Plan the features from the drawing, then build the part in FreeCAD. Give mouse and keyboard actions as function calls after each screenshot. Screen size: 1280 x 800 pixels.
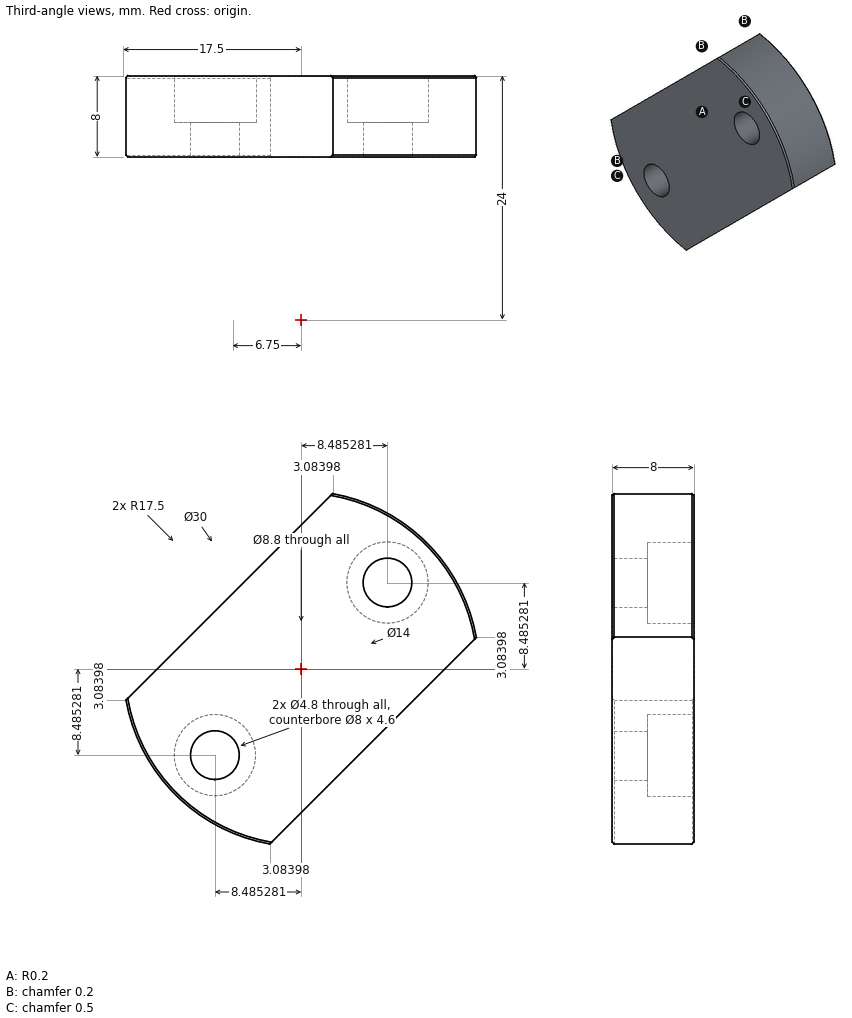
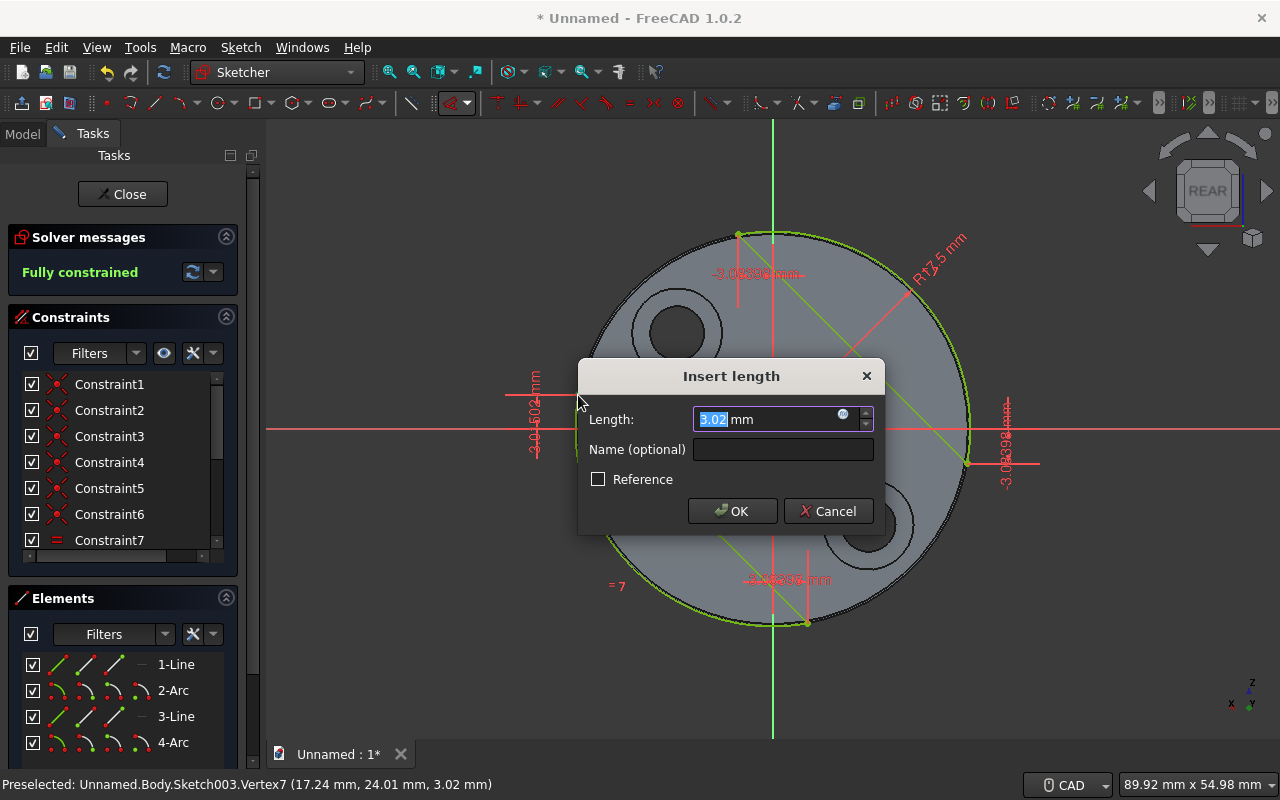
text(3.08398)
key(Return)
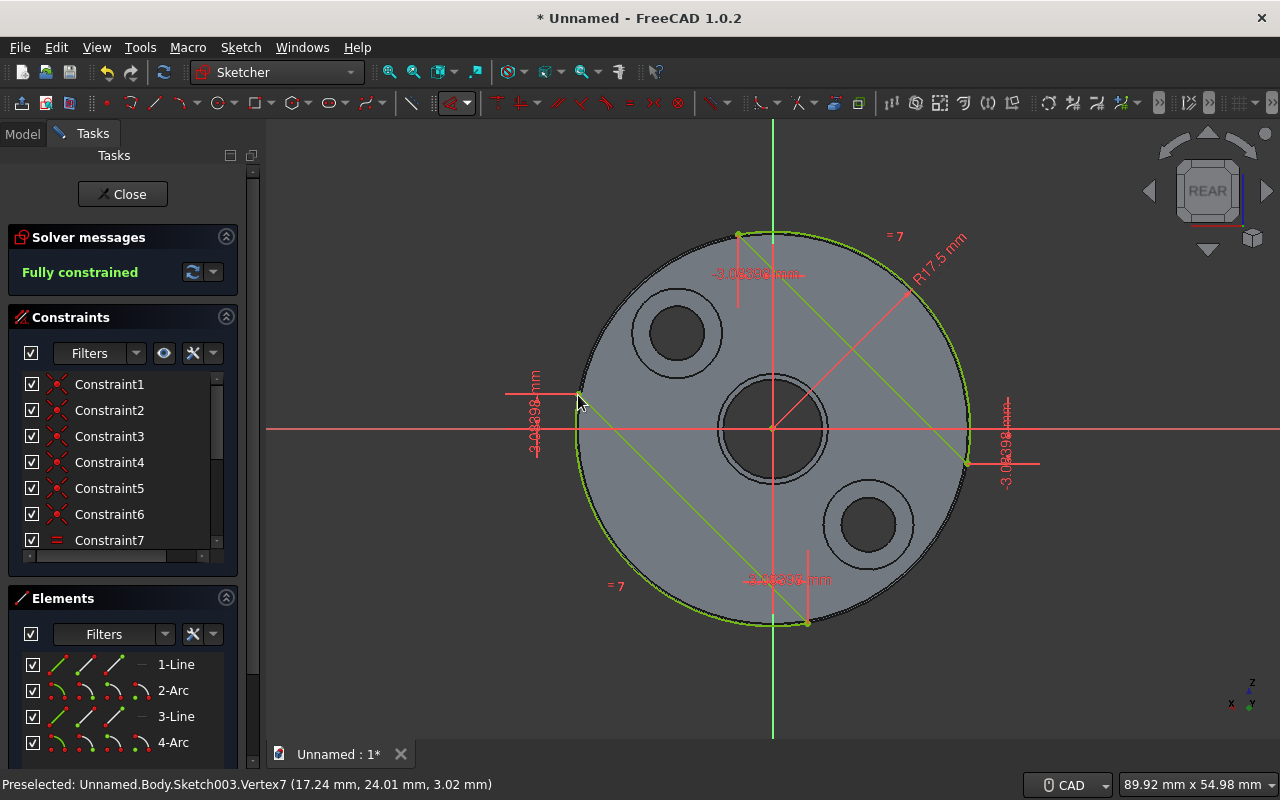
click(123, 194)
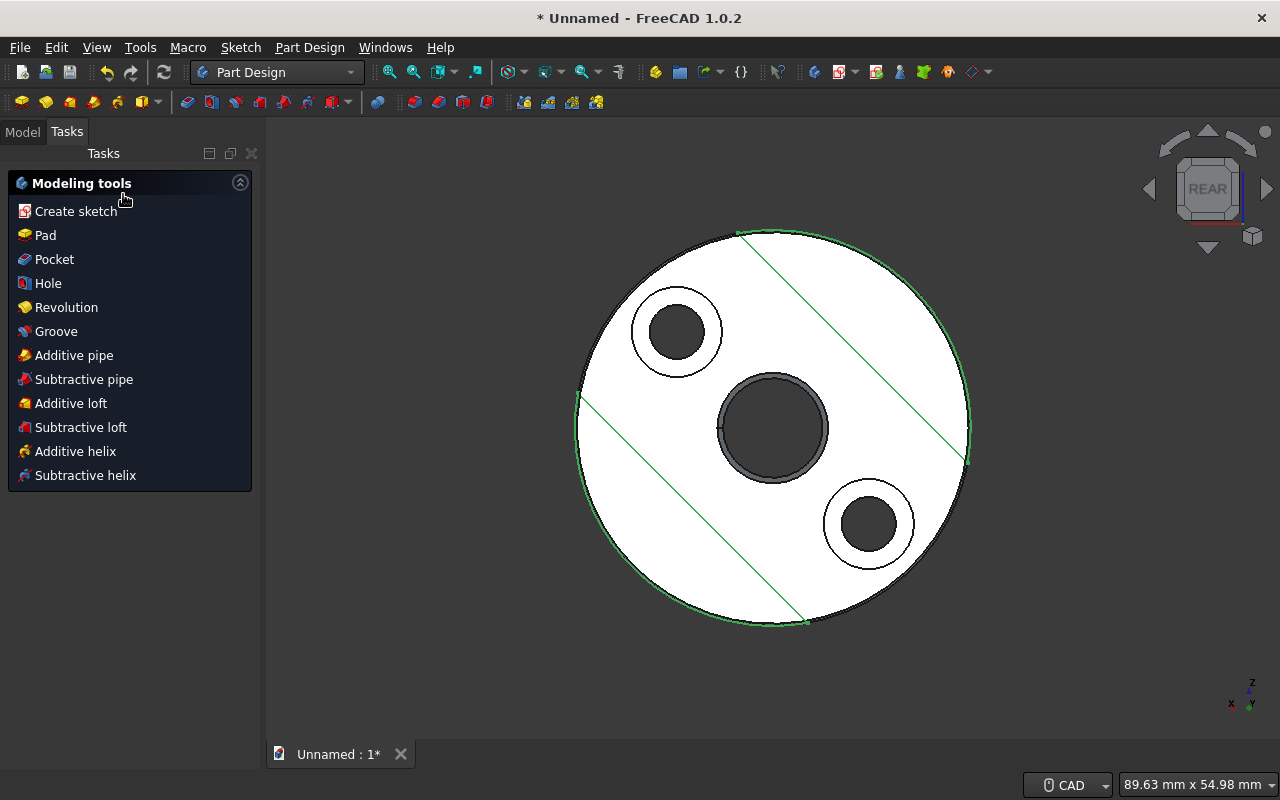
click(188, 102)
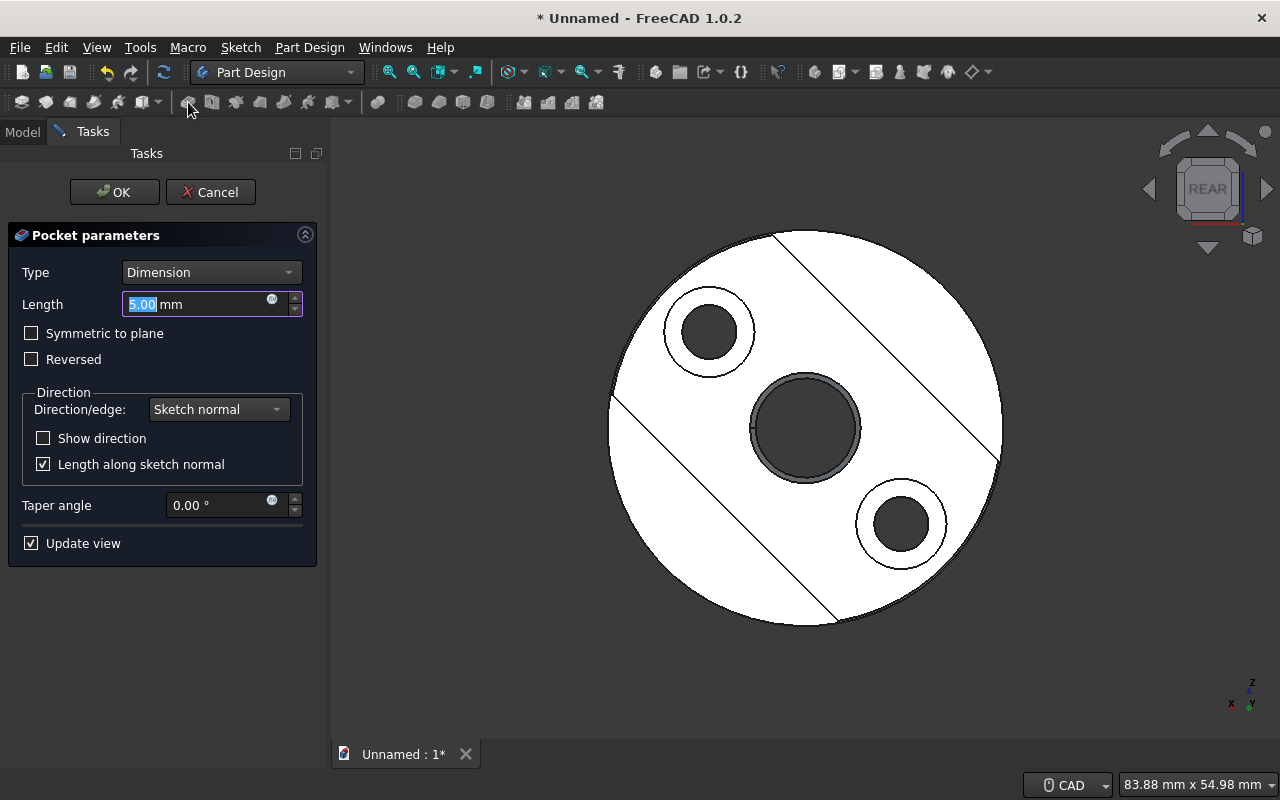
click(212, 272)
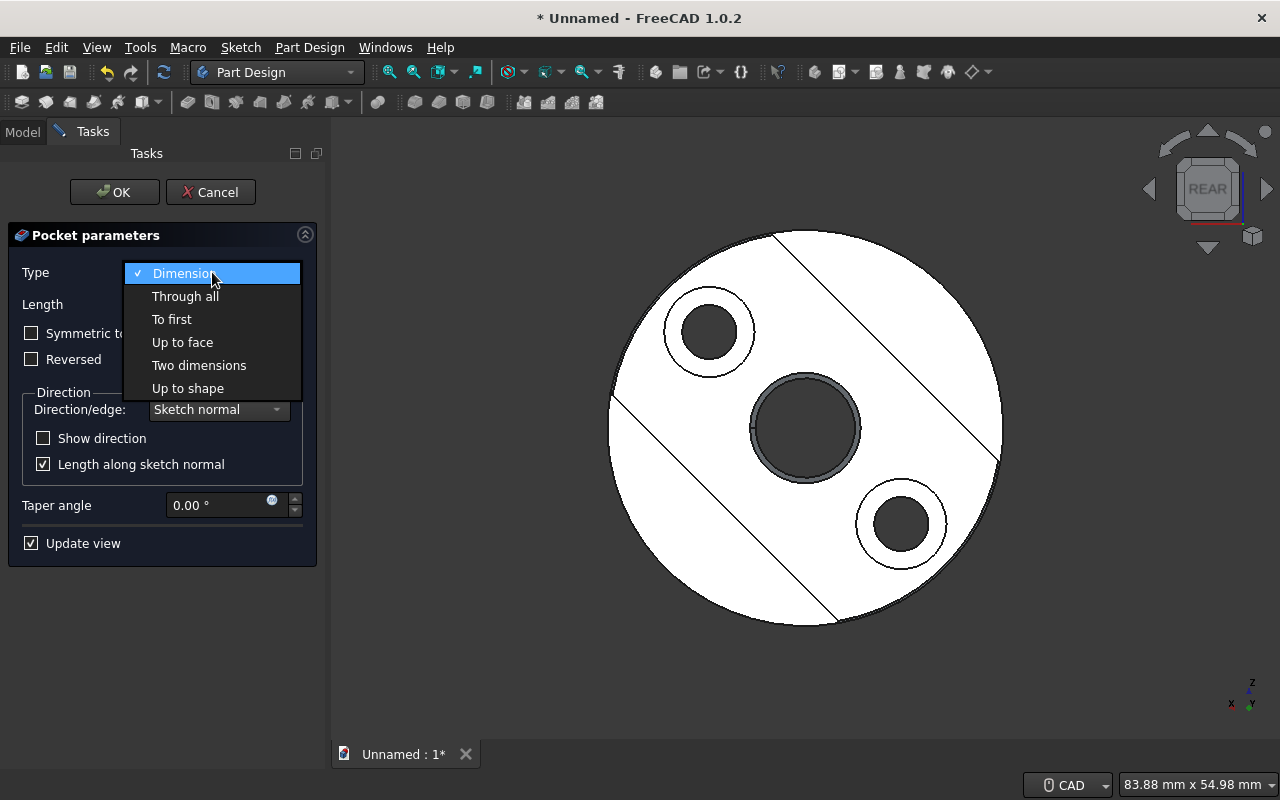
click(212, 296)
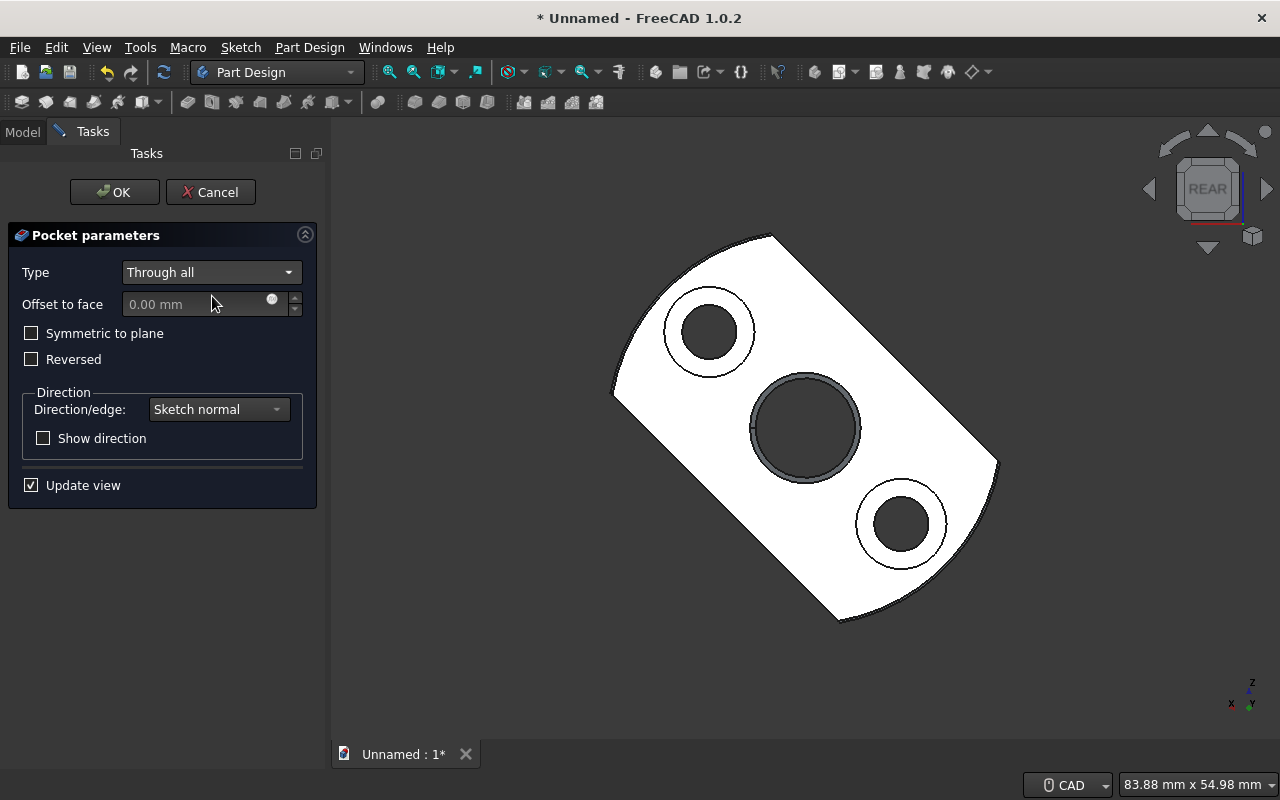
click(115, 192)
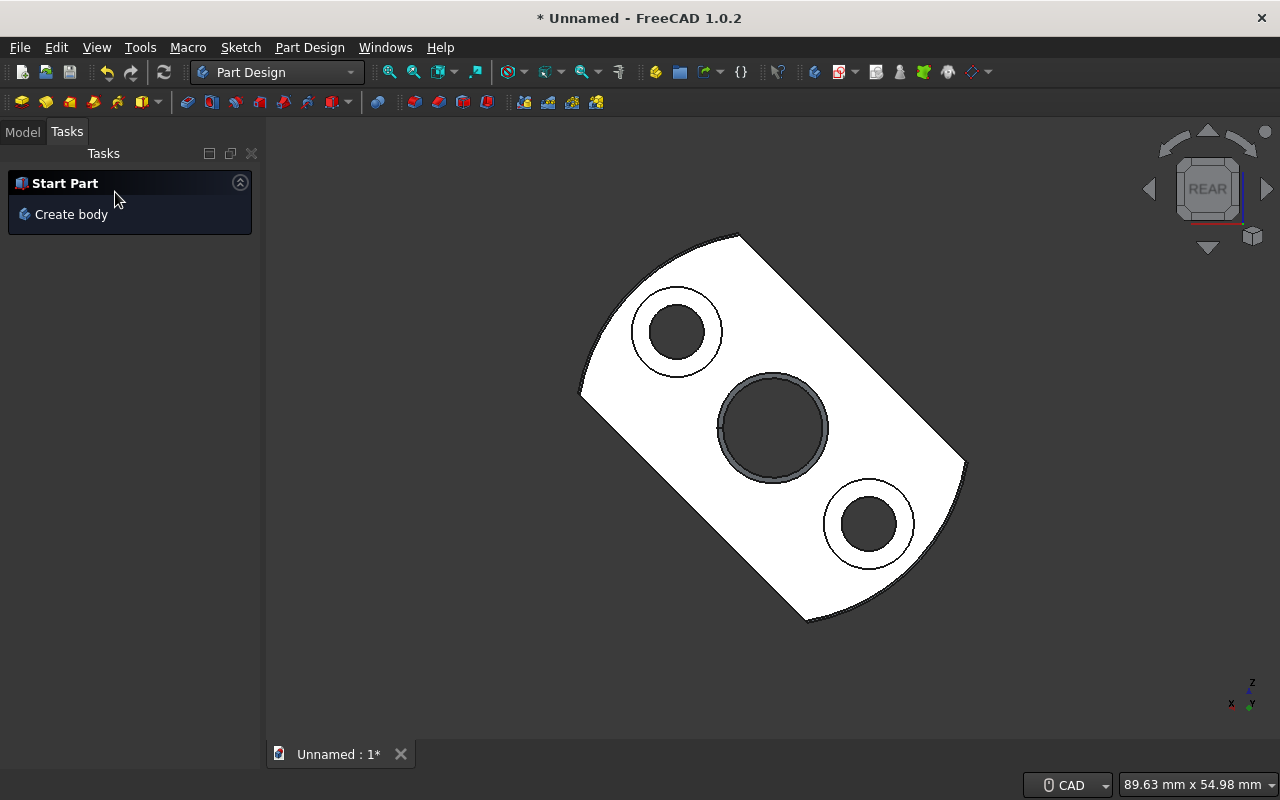
key(0)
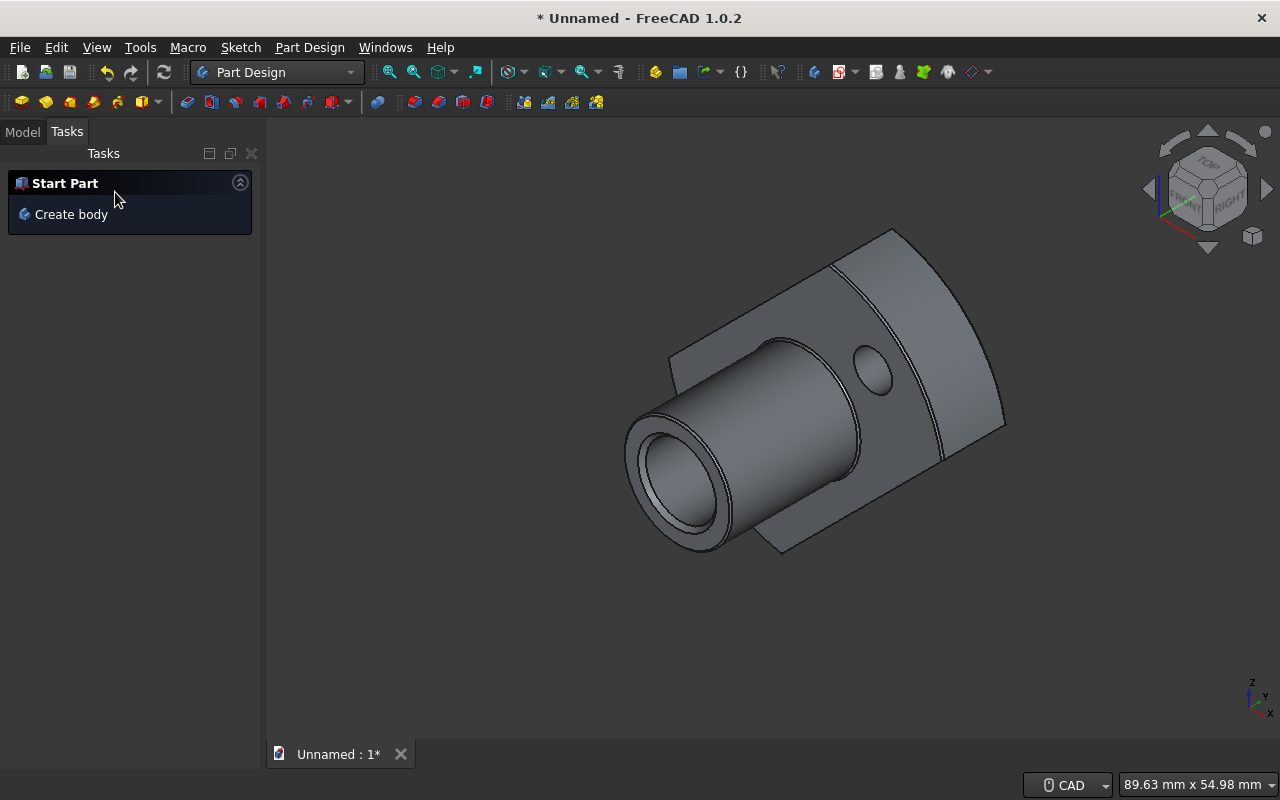
click(883, 454)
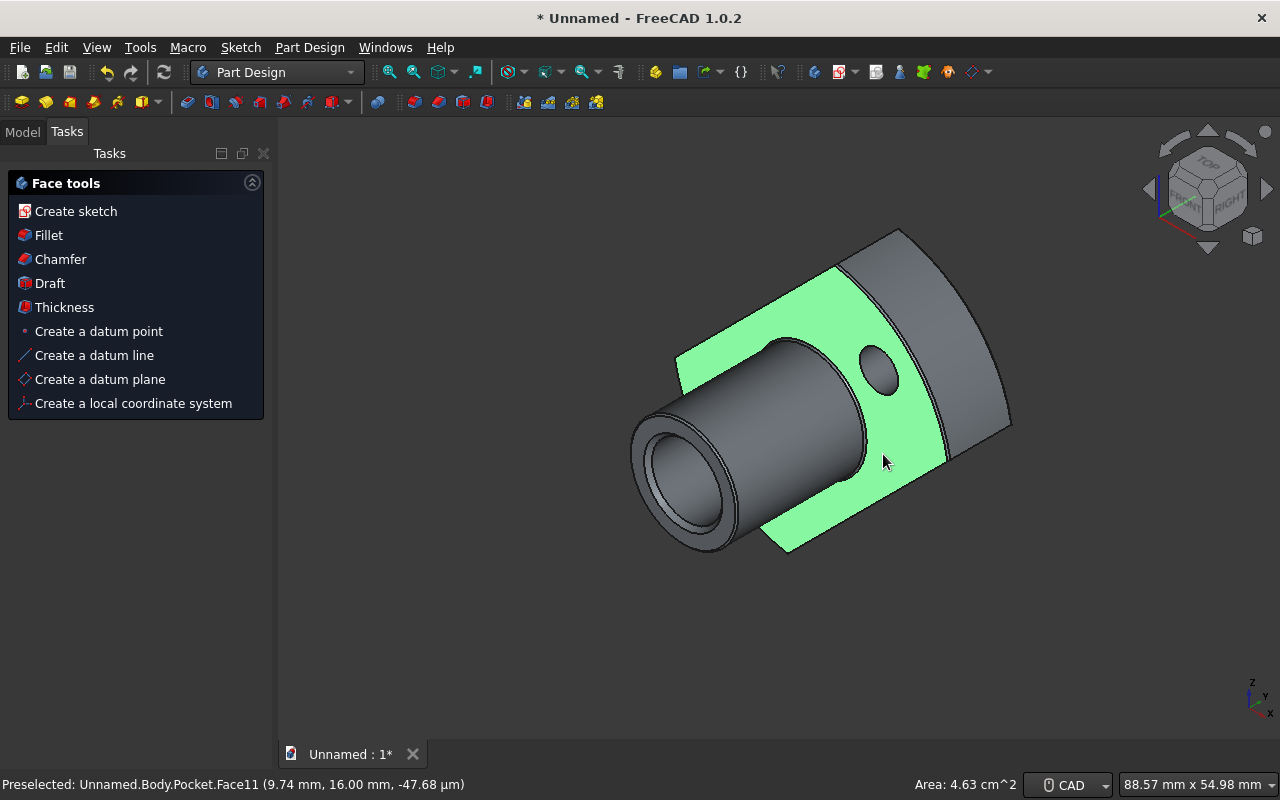
click(840, 72)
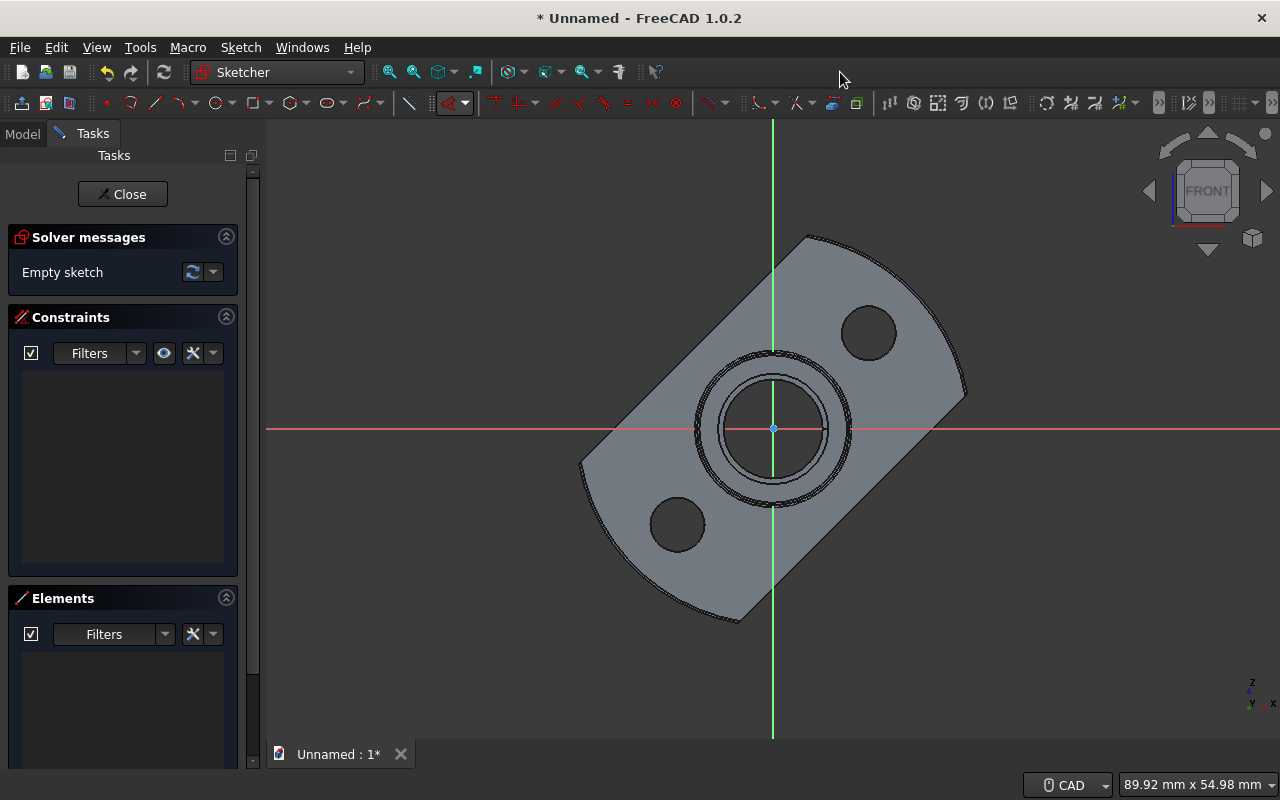
click(70, 104)